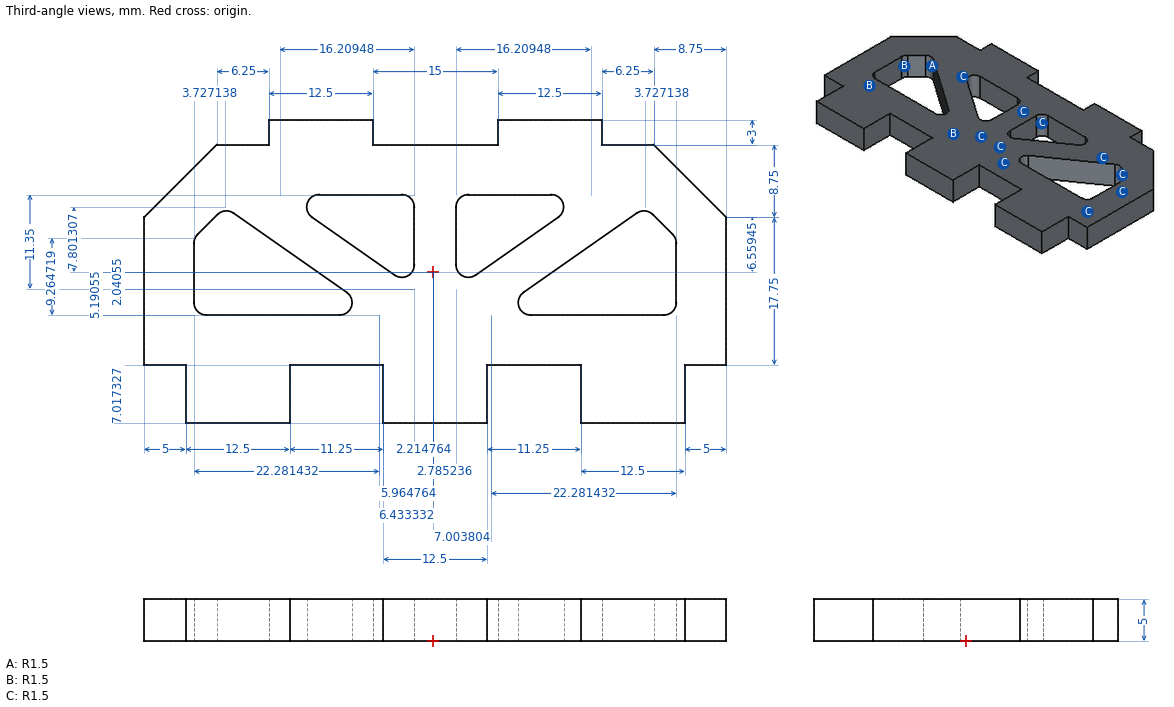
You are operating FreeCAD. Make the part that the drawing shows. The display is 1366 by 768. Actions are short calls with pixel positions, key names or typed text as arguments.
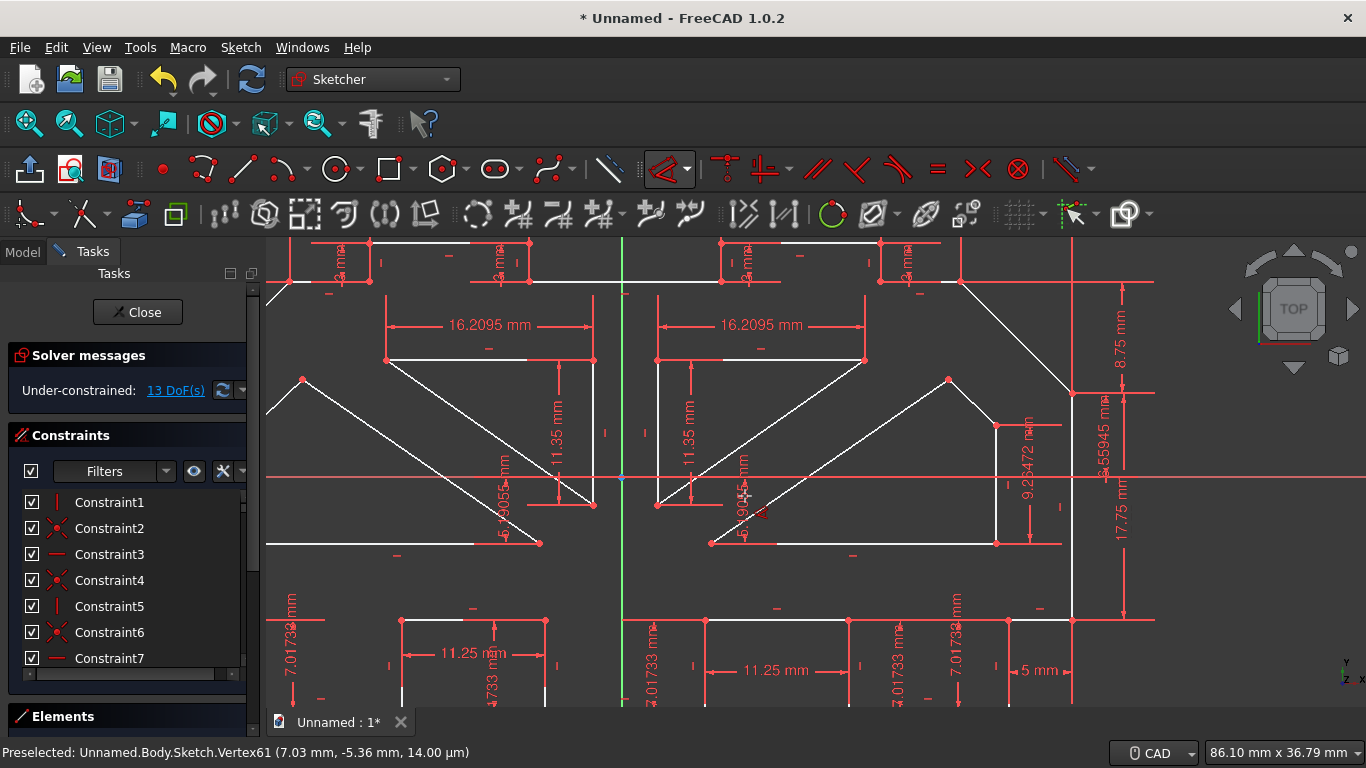
scroll(593, 505, up, 3)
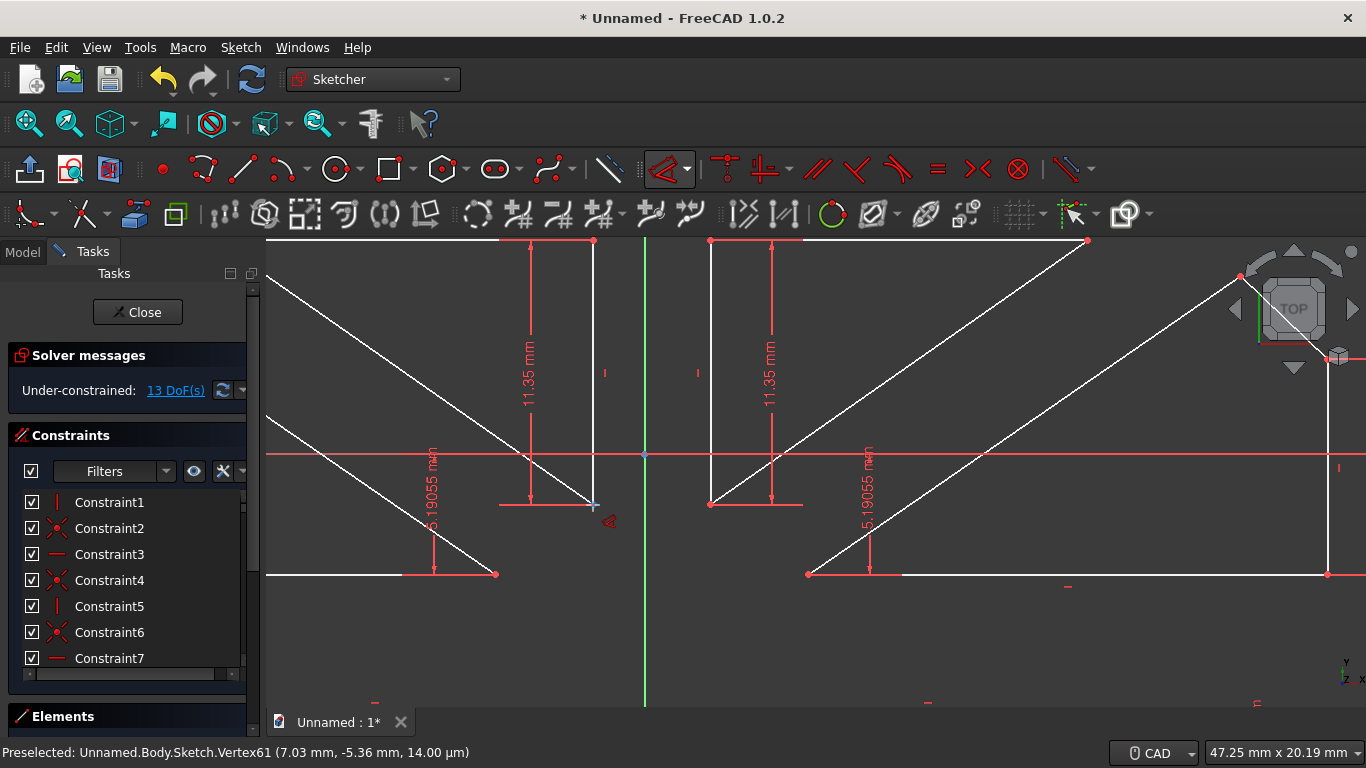
click(593, 505)
click(559, 497)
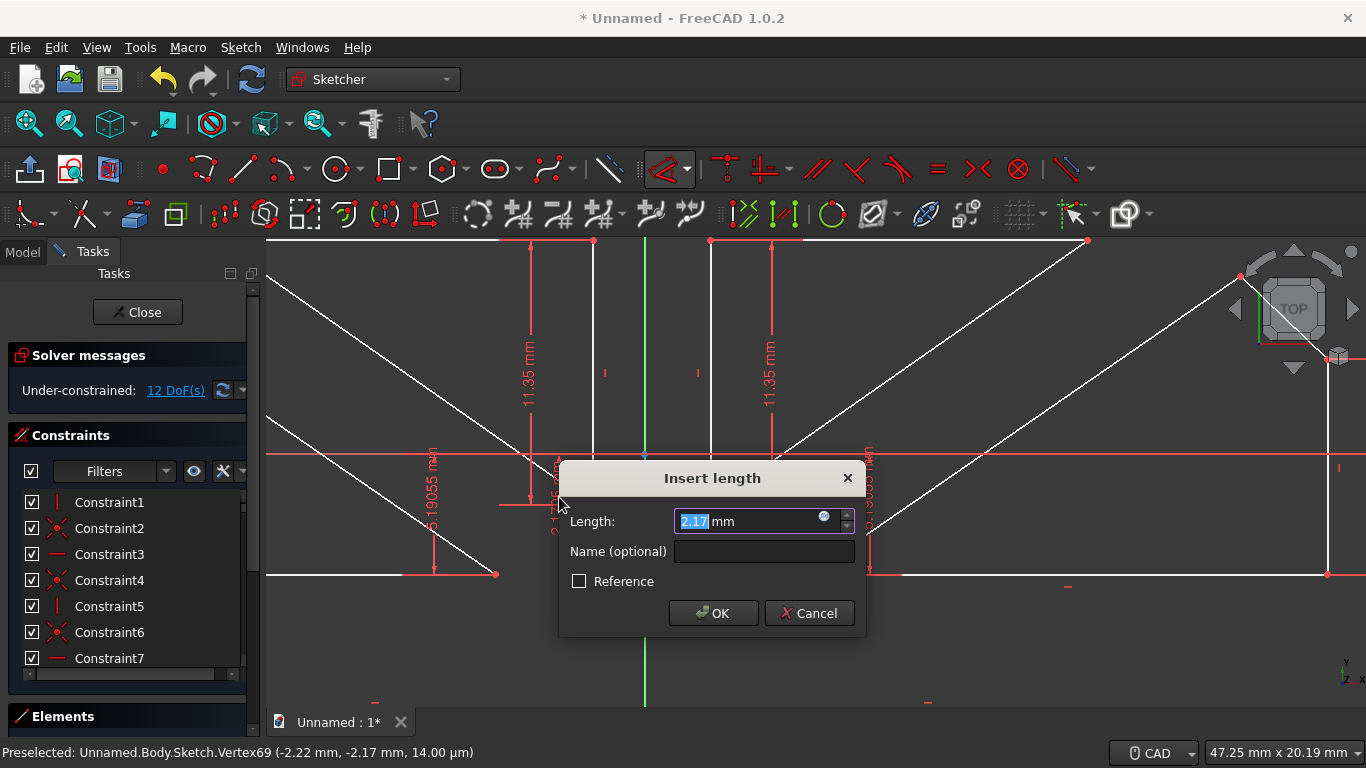
text(2.04055)
key(Return)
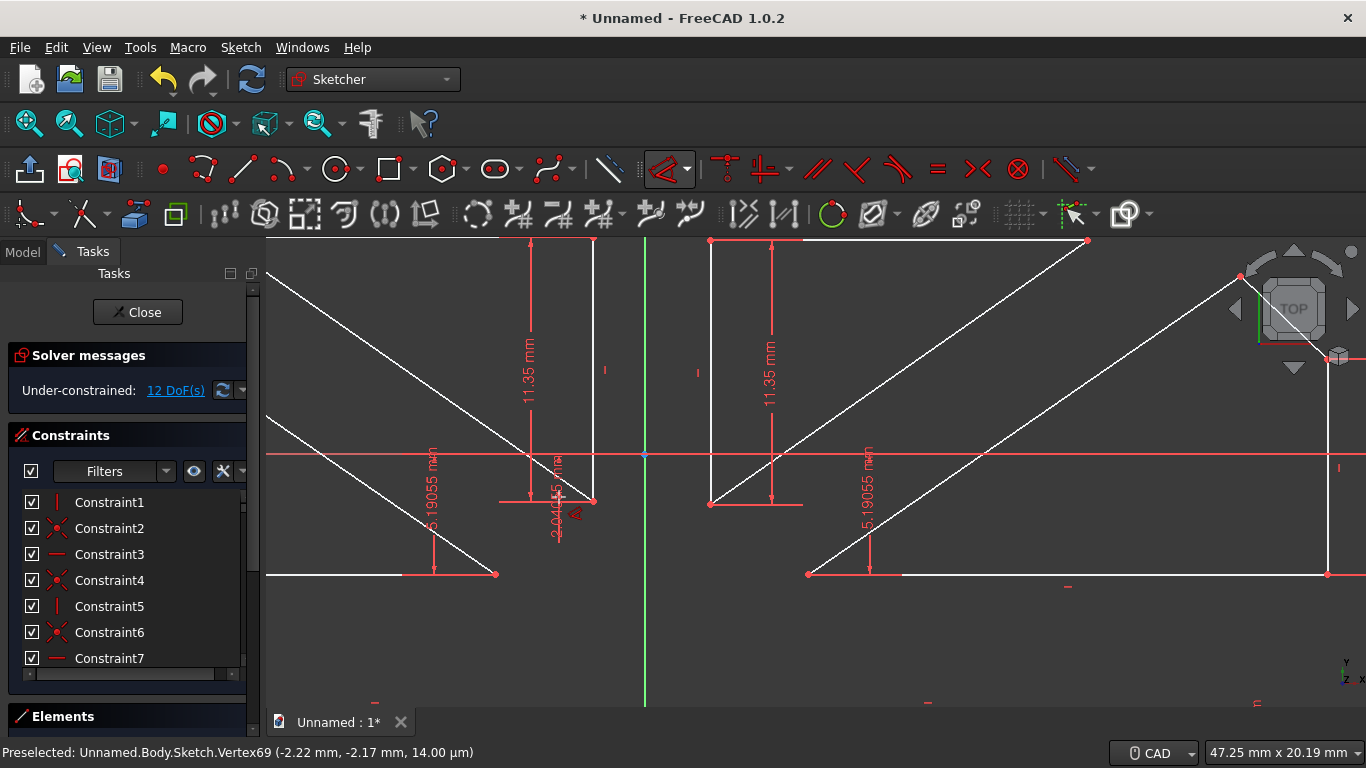
click(711, 505)
click(745, 497)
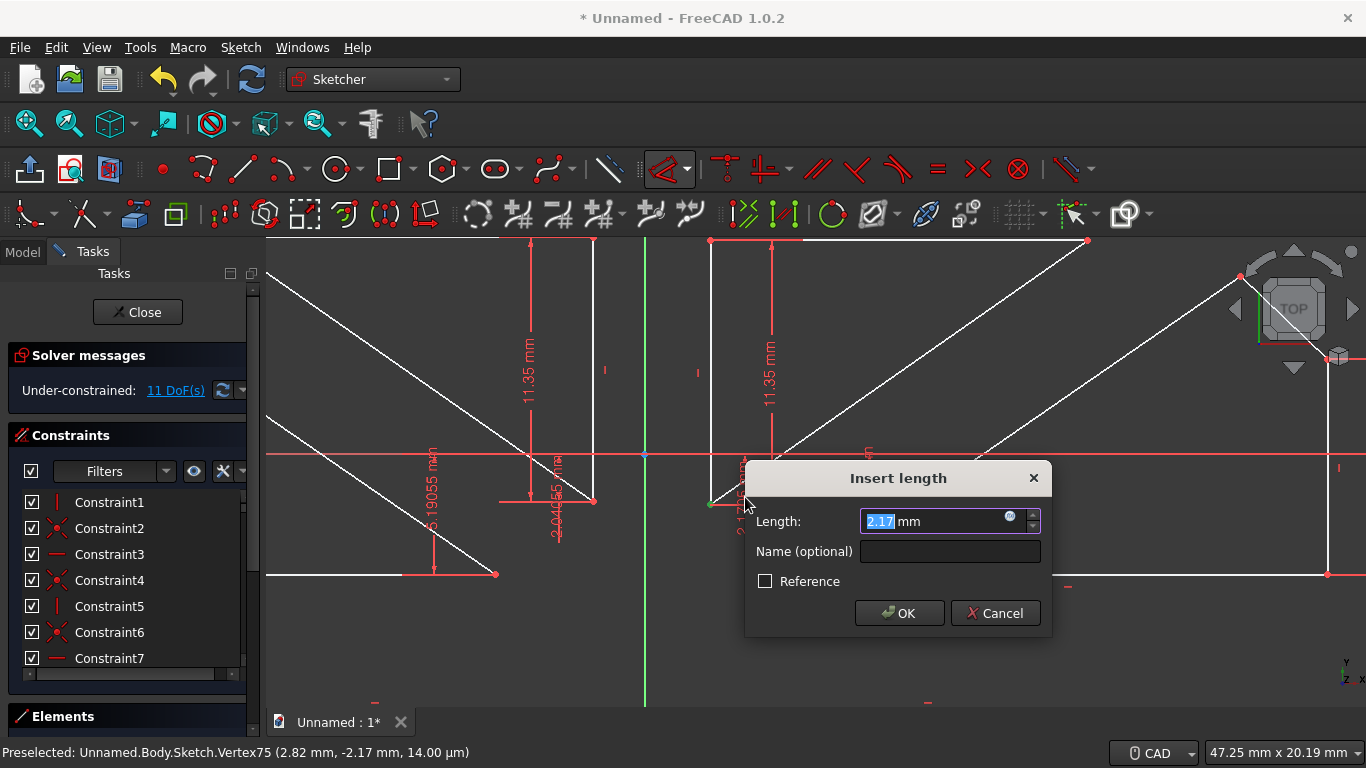
text(2.04055)
key(Return)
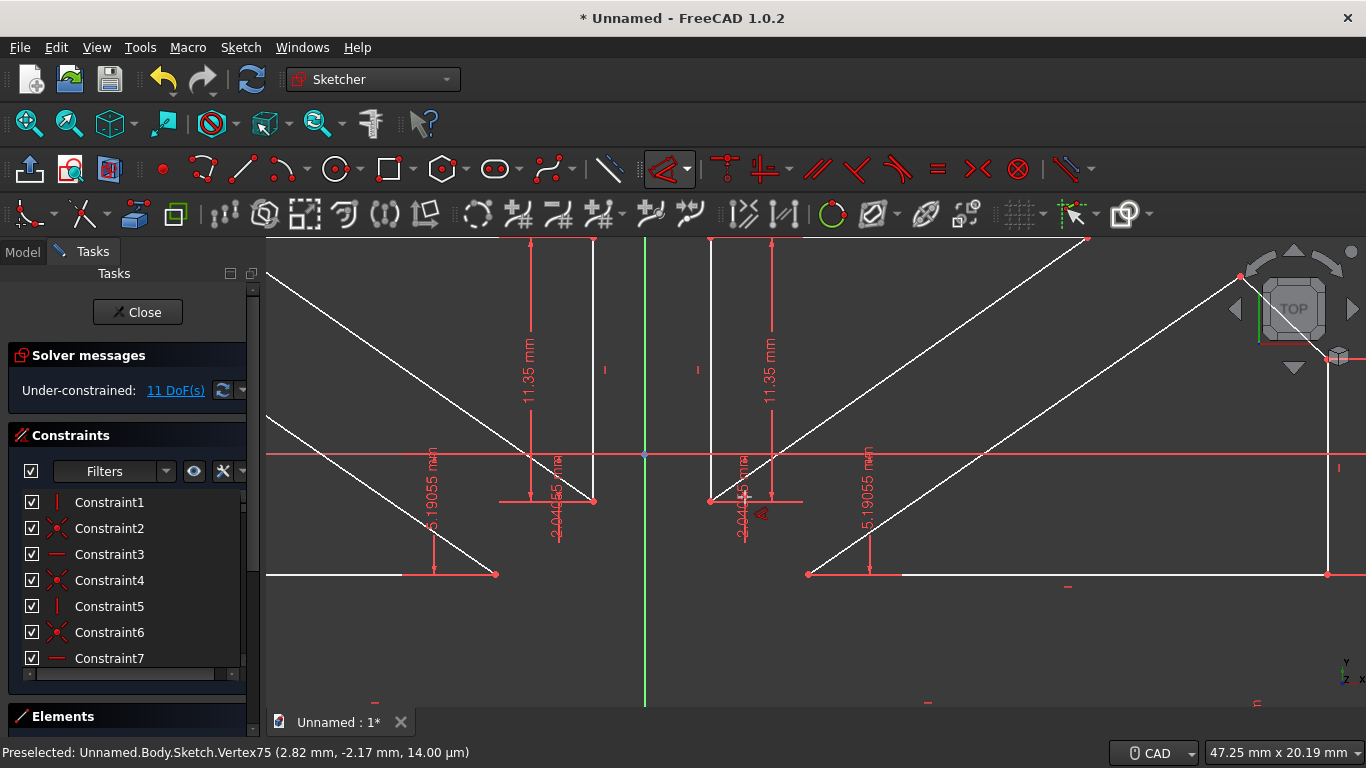
click(340, 575)
click(395, 609)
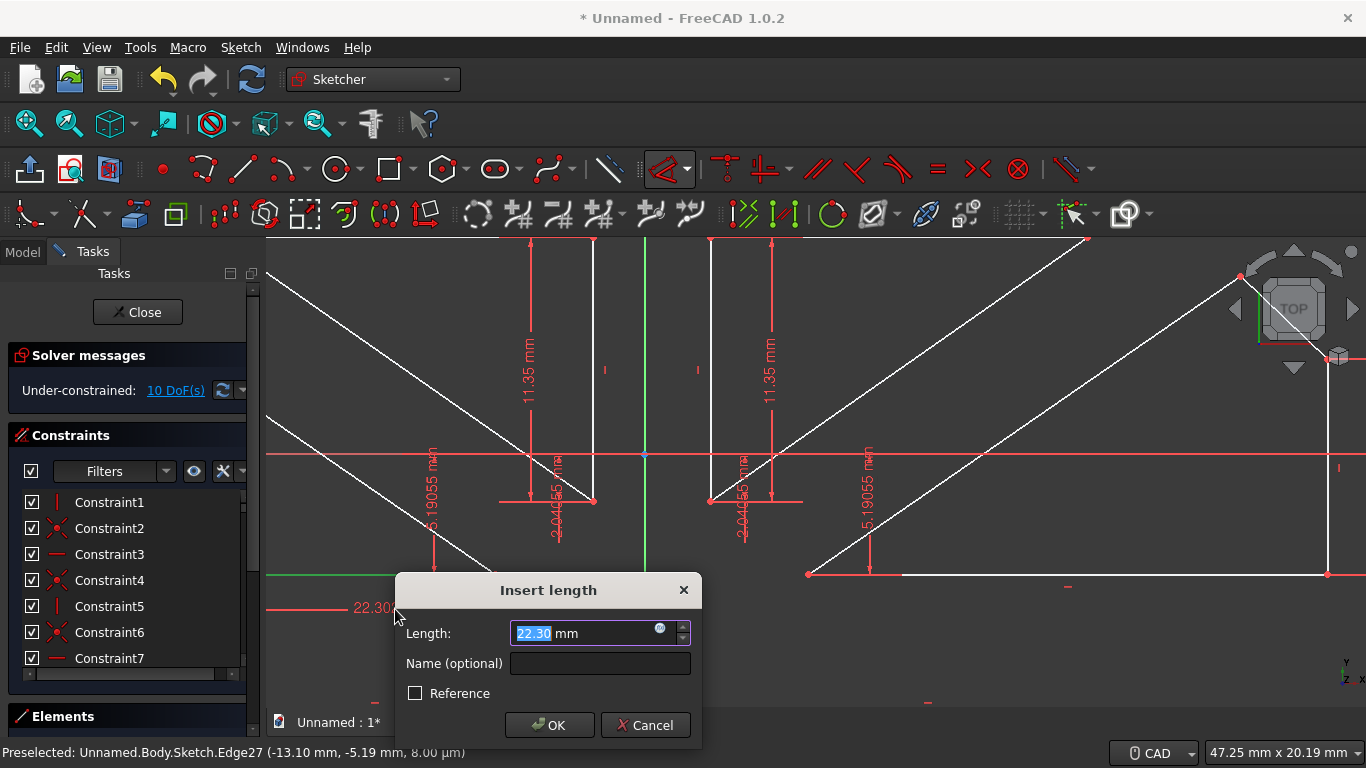
text(22.281432)
key(Return)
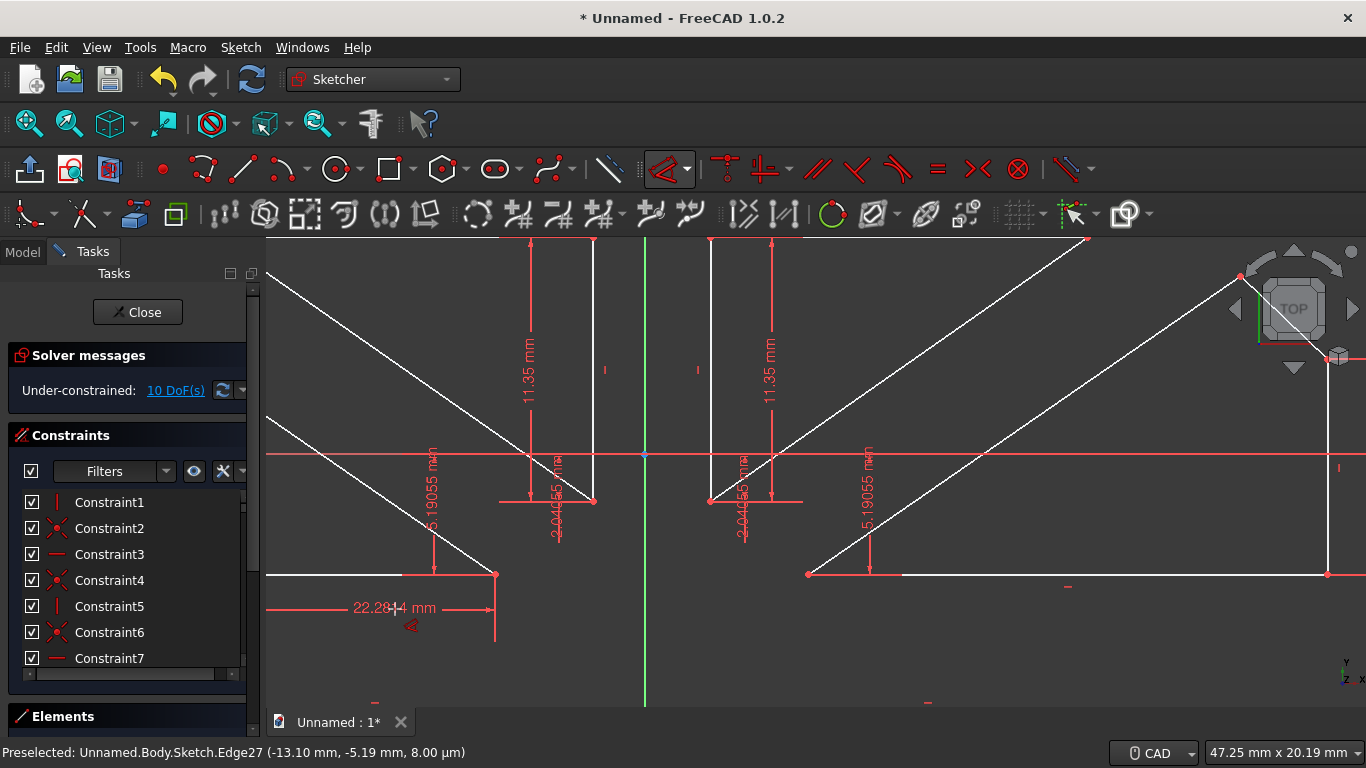
click(1172, 575)
click(1005, 609)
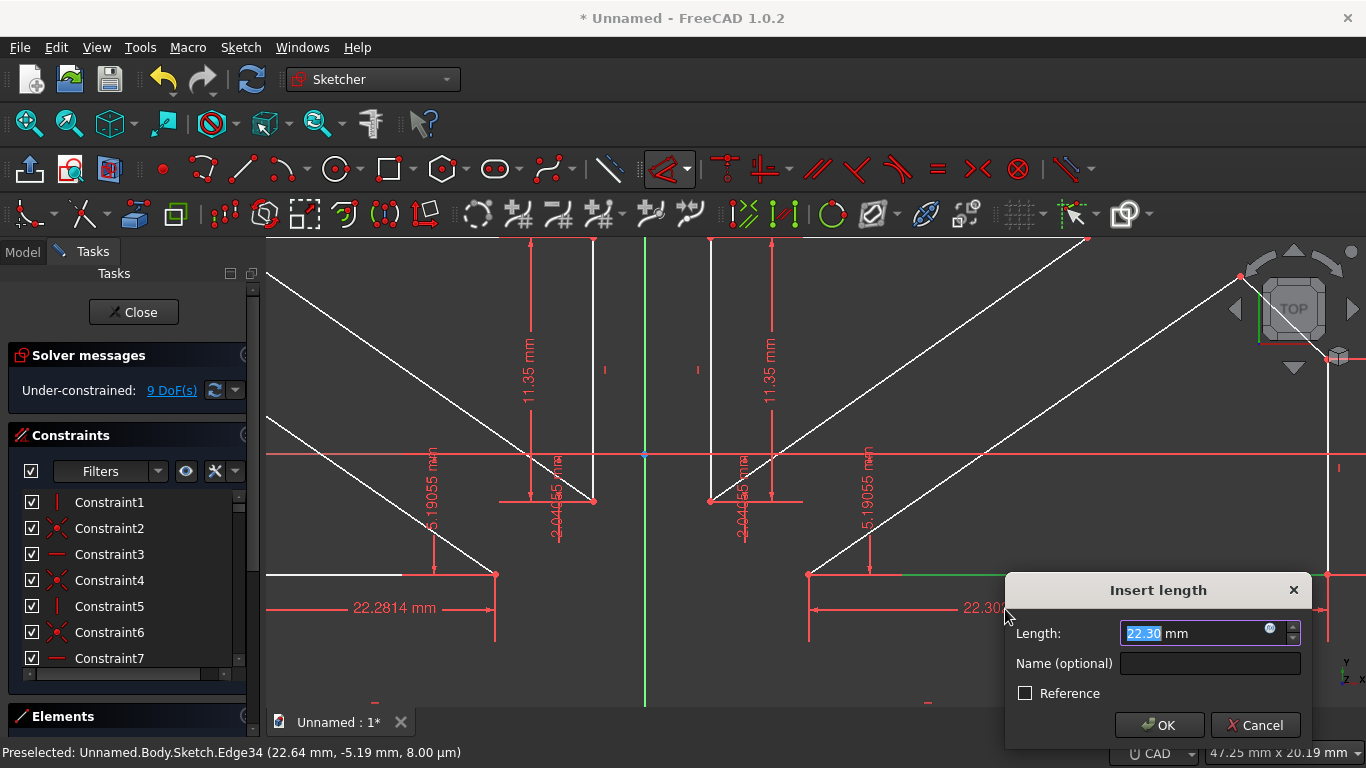
text(22.281432)
key(Return)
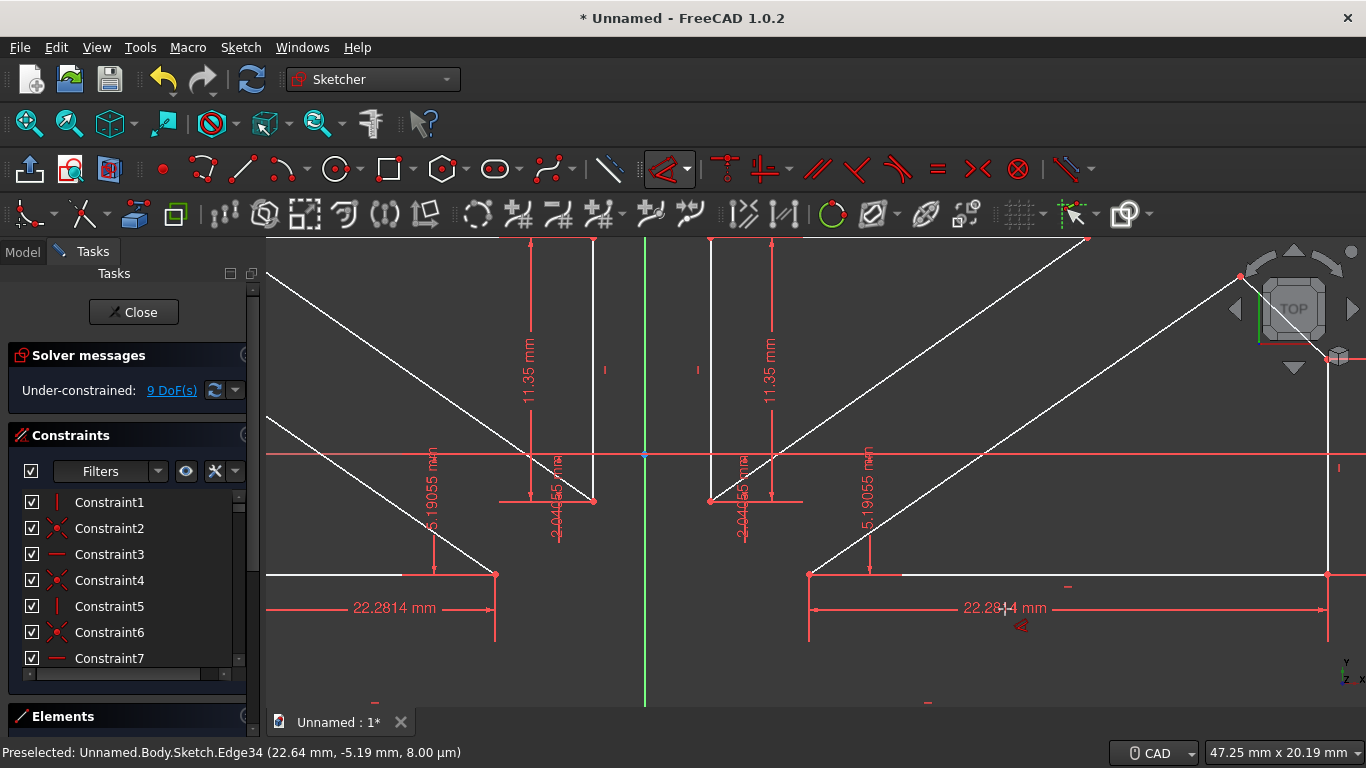
scroll(803, 483, down, 5)